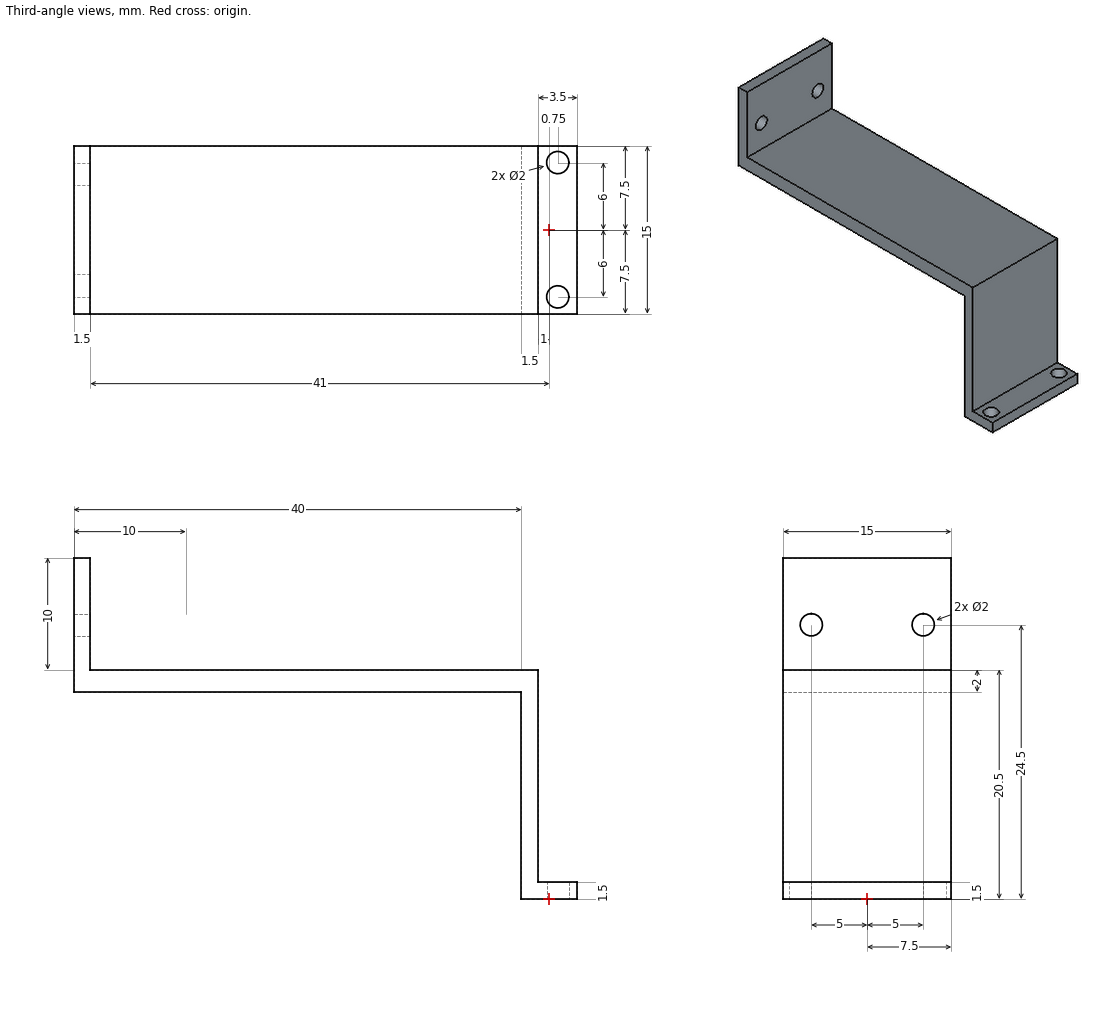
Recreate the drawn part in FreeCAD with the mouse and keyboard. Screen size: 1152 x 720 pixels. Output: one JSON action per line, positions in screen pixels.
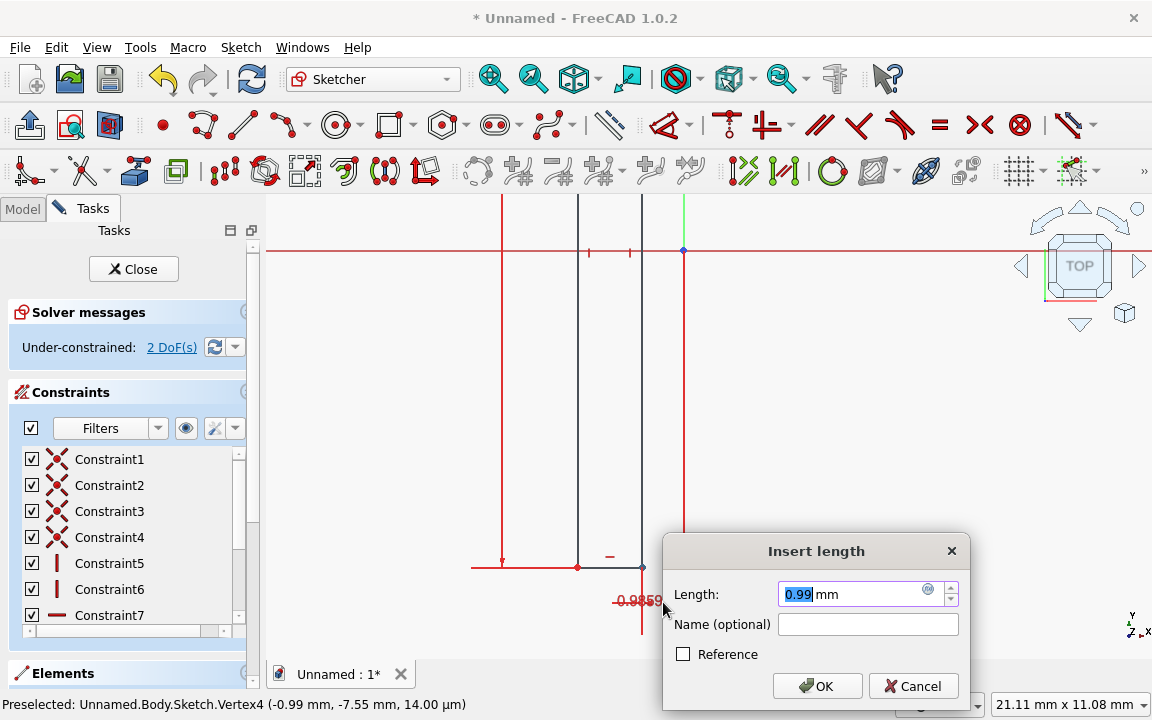
{"action": "type", "text": "1"}
{"action": "key", "text": "Return"}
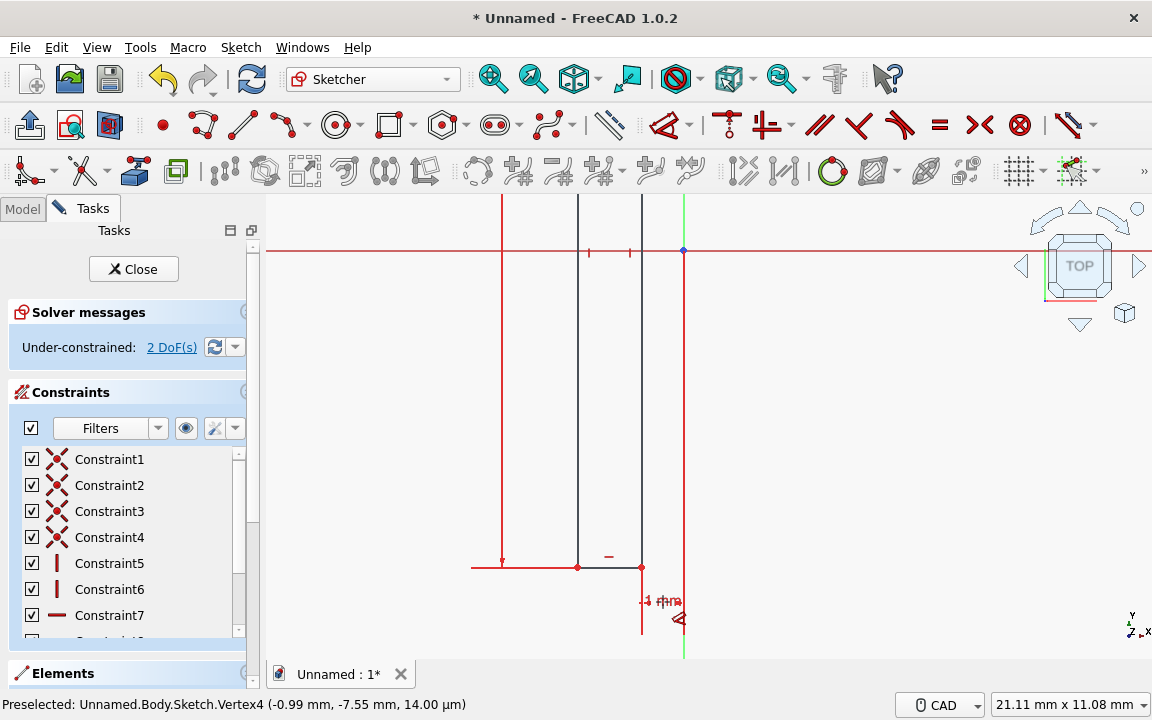
{"action": "left_click", "coordinate": [597, 568]}
{"action": "left_click", "coordinate": [588, 602]}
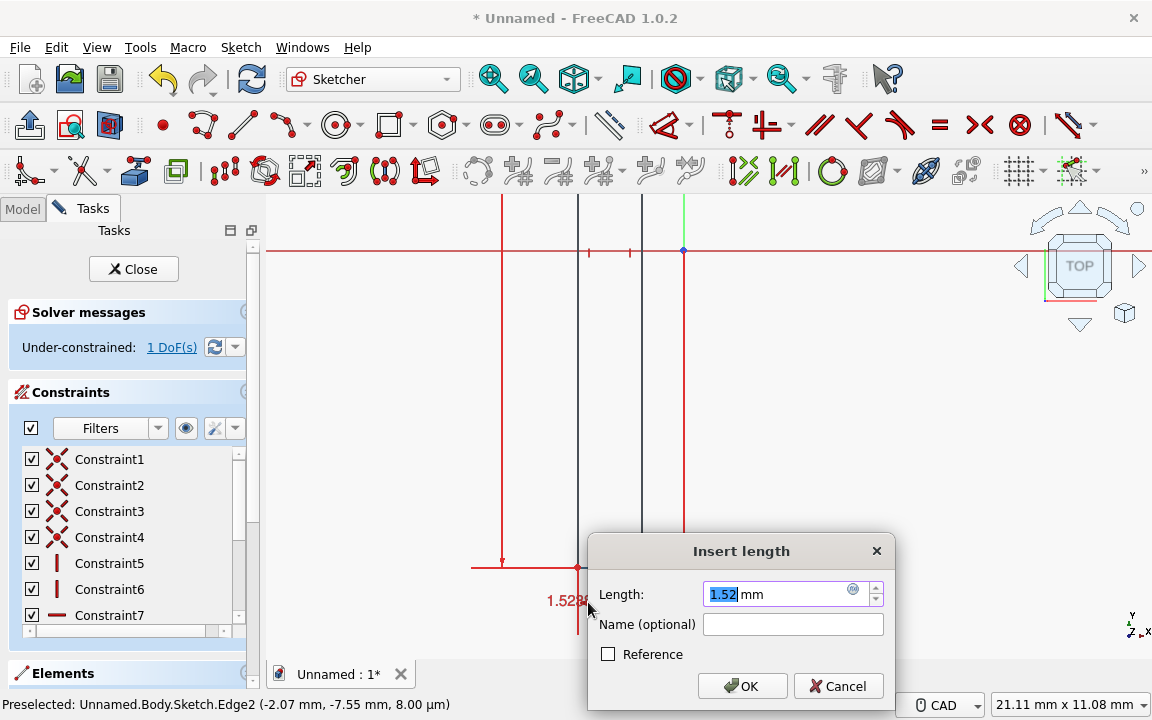
{"action": "type", "text": "1.5"}
{"action": "key", "text": "Return"}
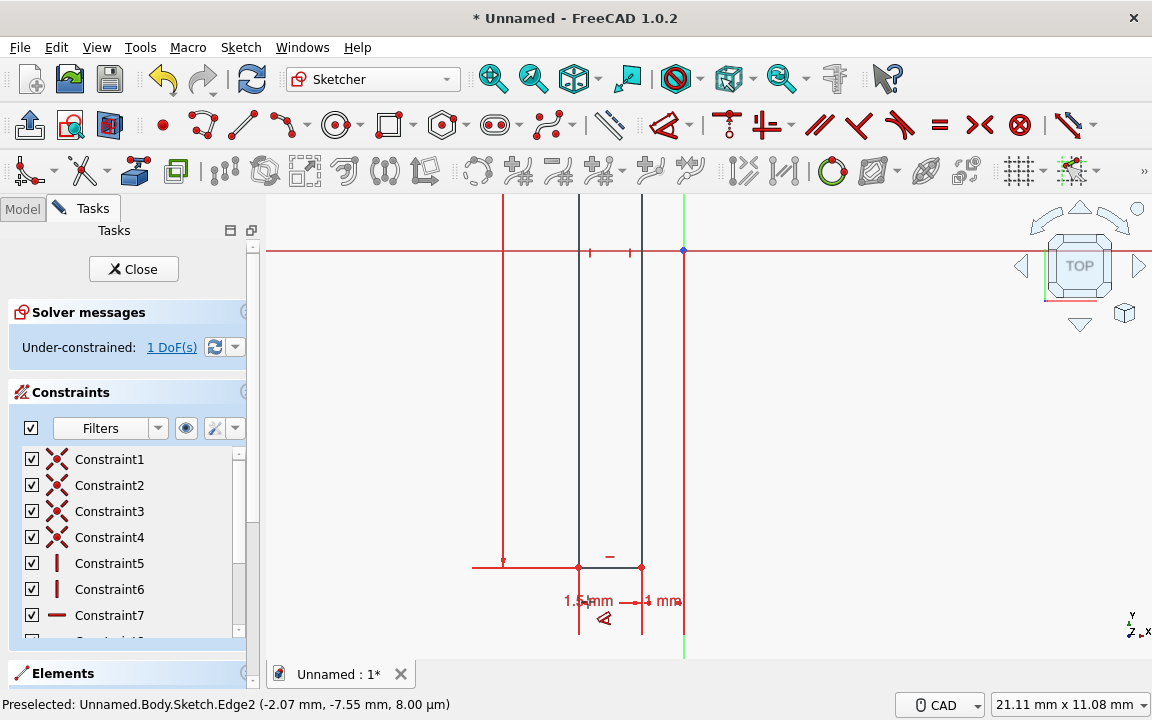
{"action": "scroll", "coordinate": [648, 570], "scroll_direction": "down", "scroll_amount": 4}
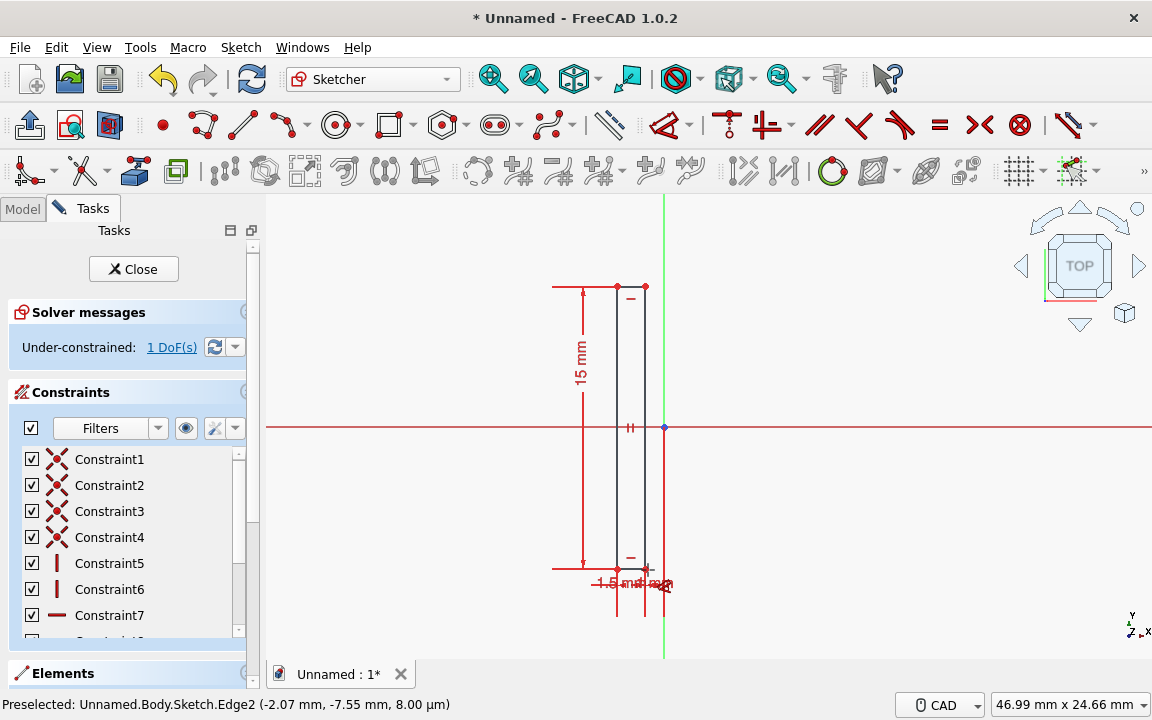
{"action": "left_click", "coordinate": [617, 287]}
{"action": "left_click", "coordinate": [698, 357]}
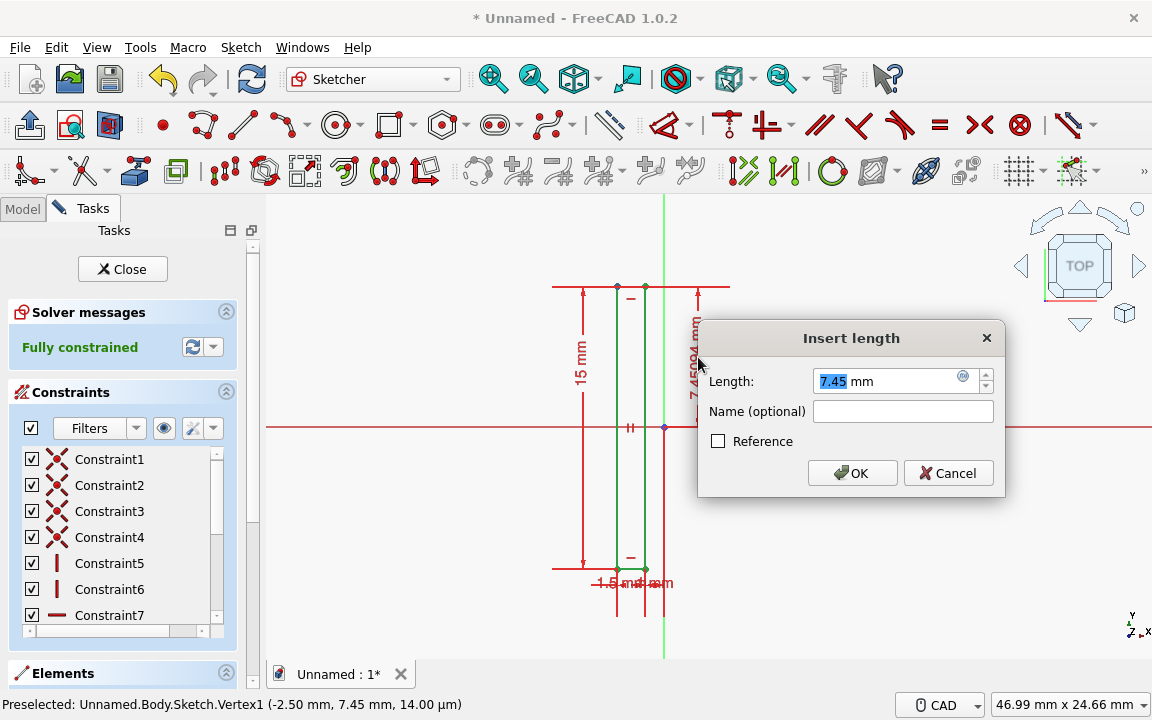
{"action": "type", "text": "7.5"}
{"action": "key", "text": "Return"}
{"action": "key", "text": "Escape"}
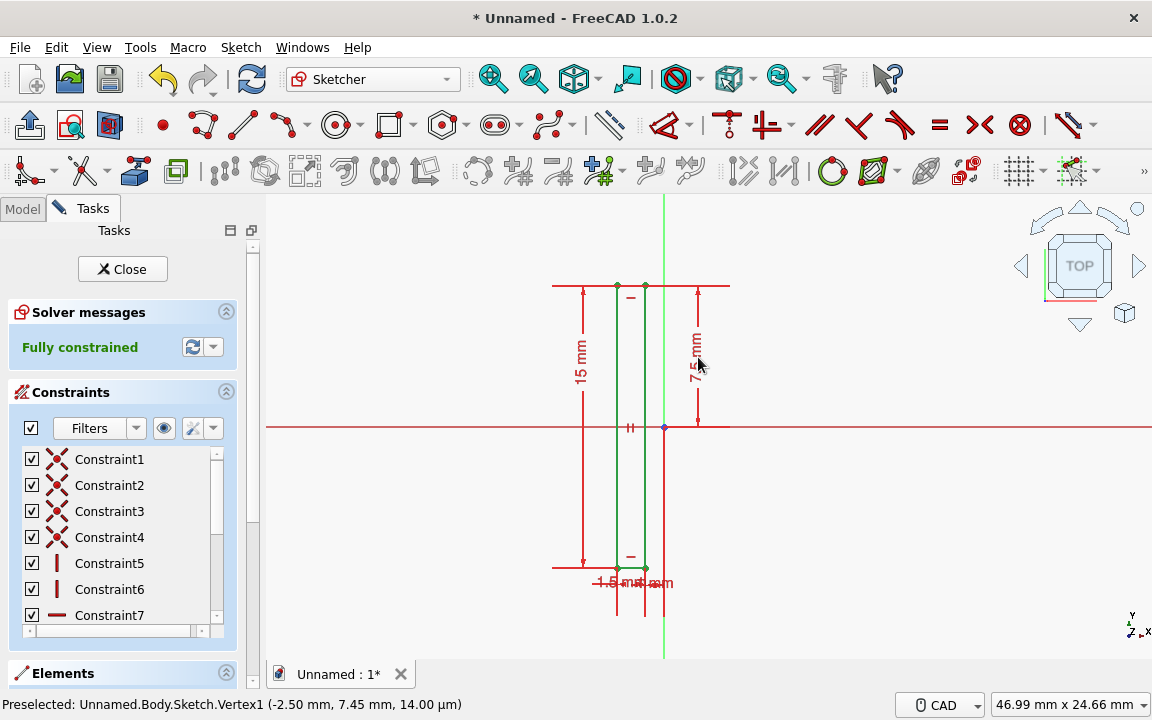
{"action": "left_click", "coordinate": [123, 269]}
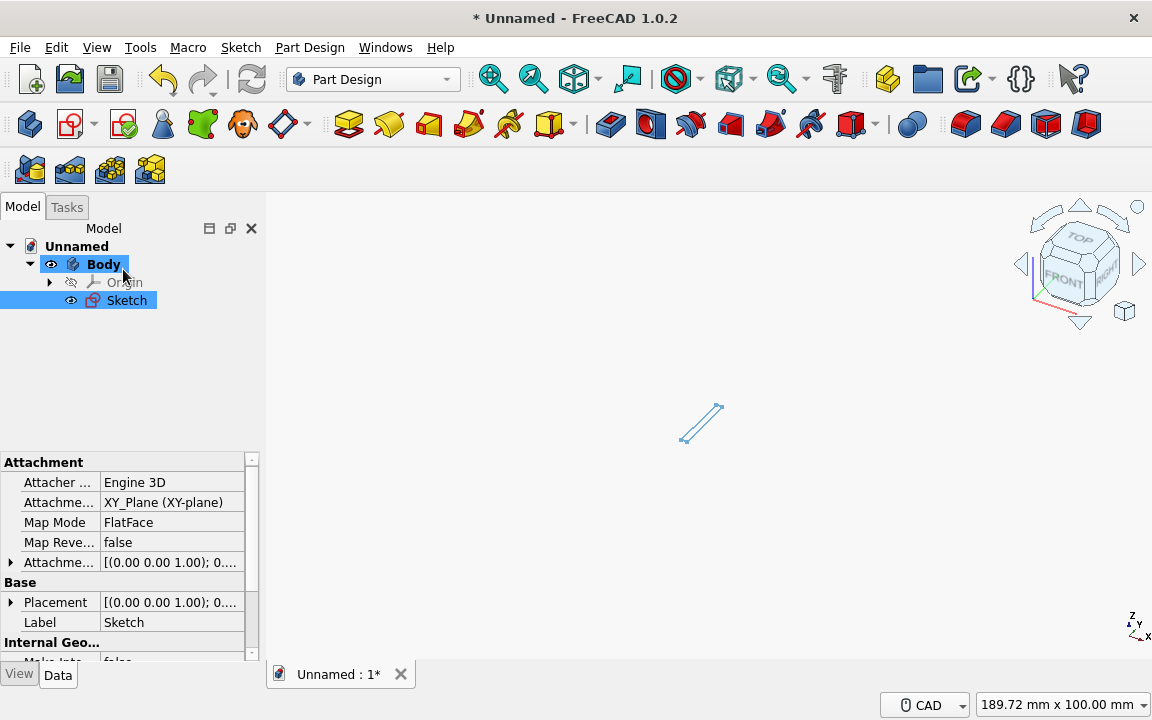
{"action": "left_click", "coordinate": [350, 124]}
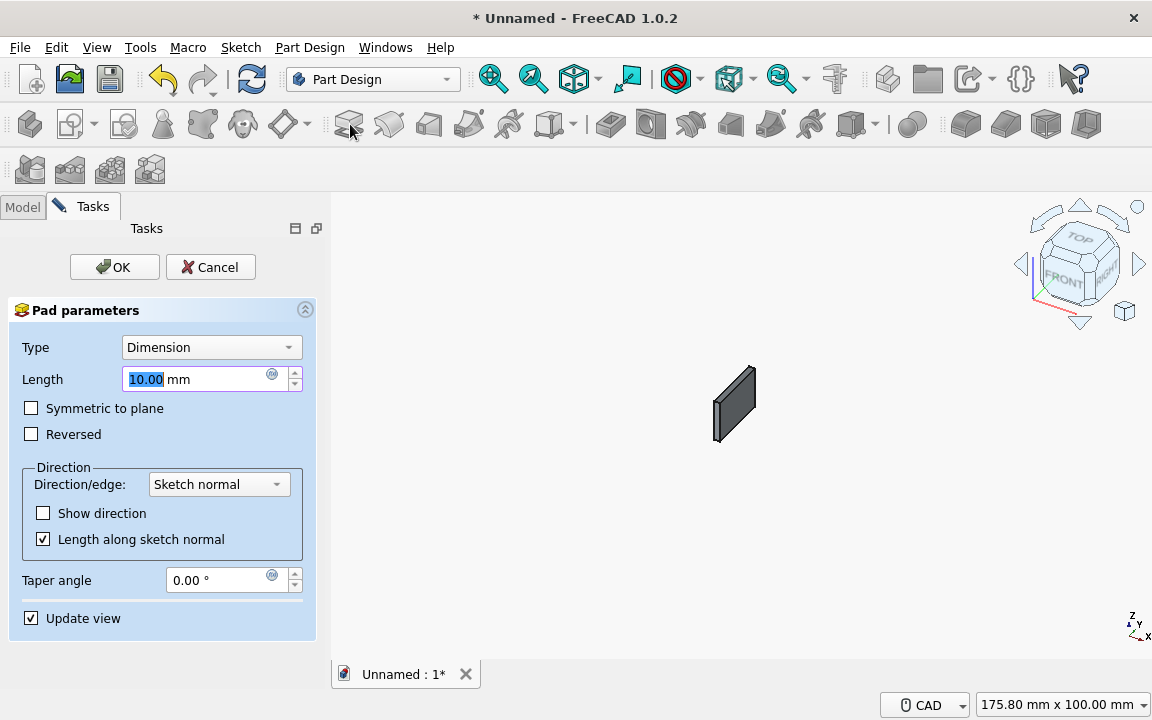
{"action": "type", "text": "20.5"}
{"action": "key", "text": "Tab"}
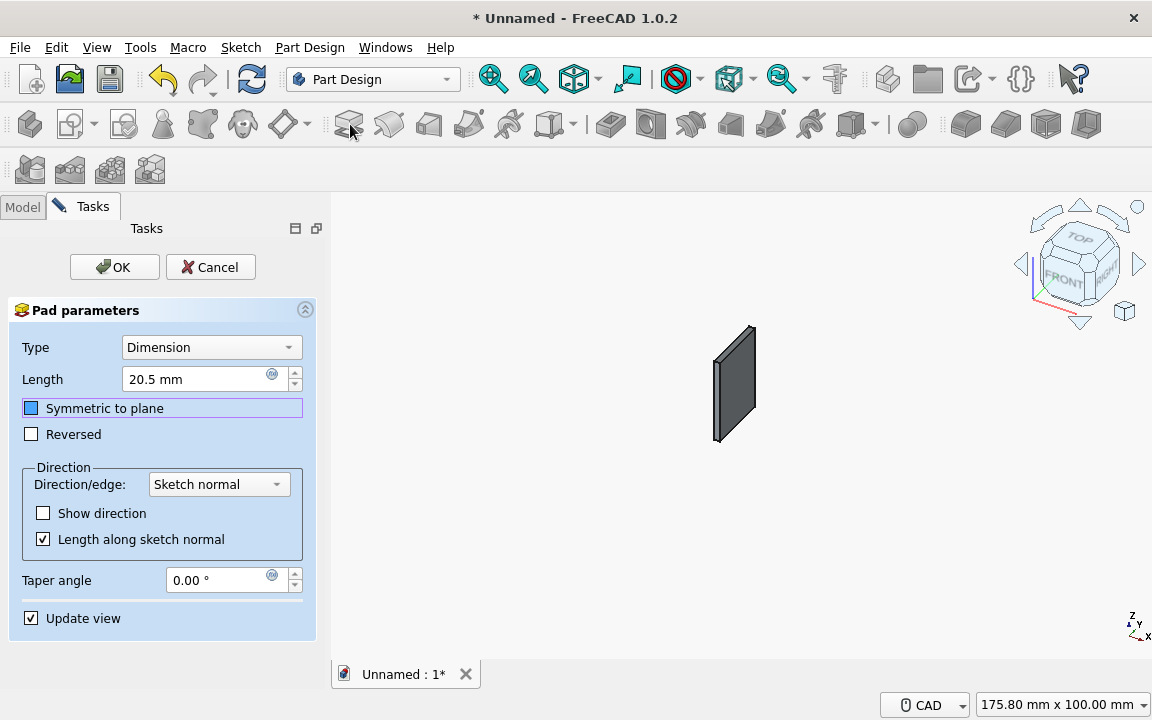
{"action": "left_click", "coordinate": [115, 267]}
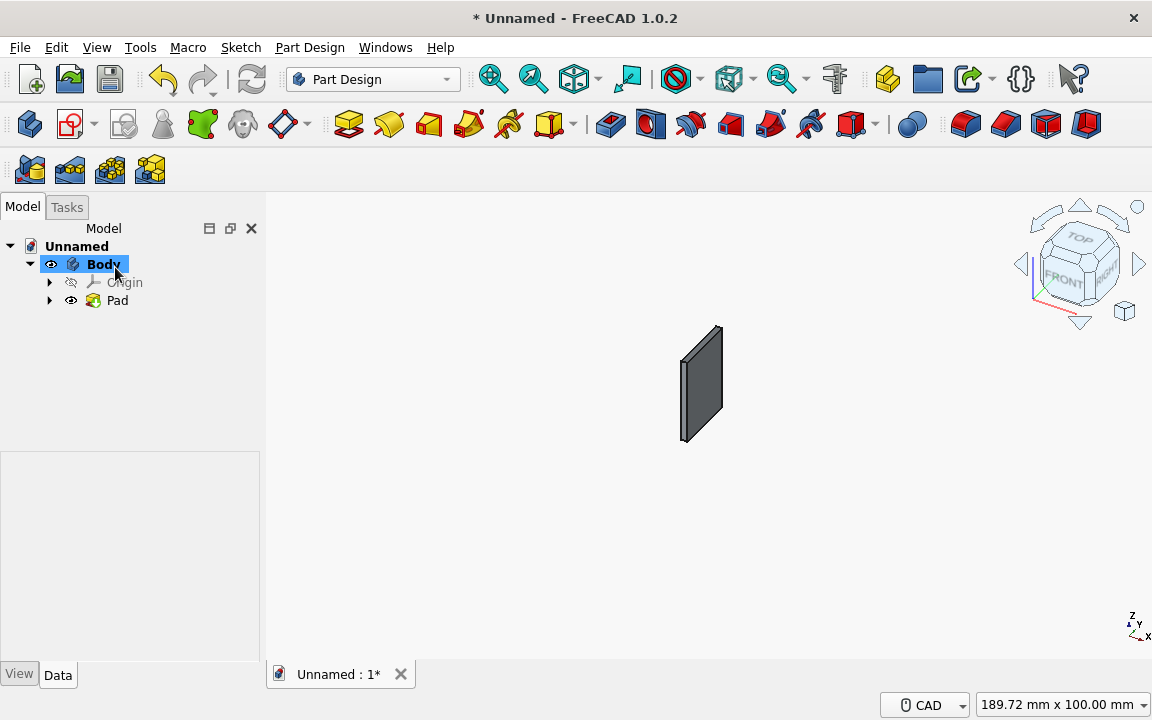
{"action": "key", "text": "v f"}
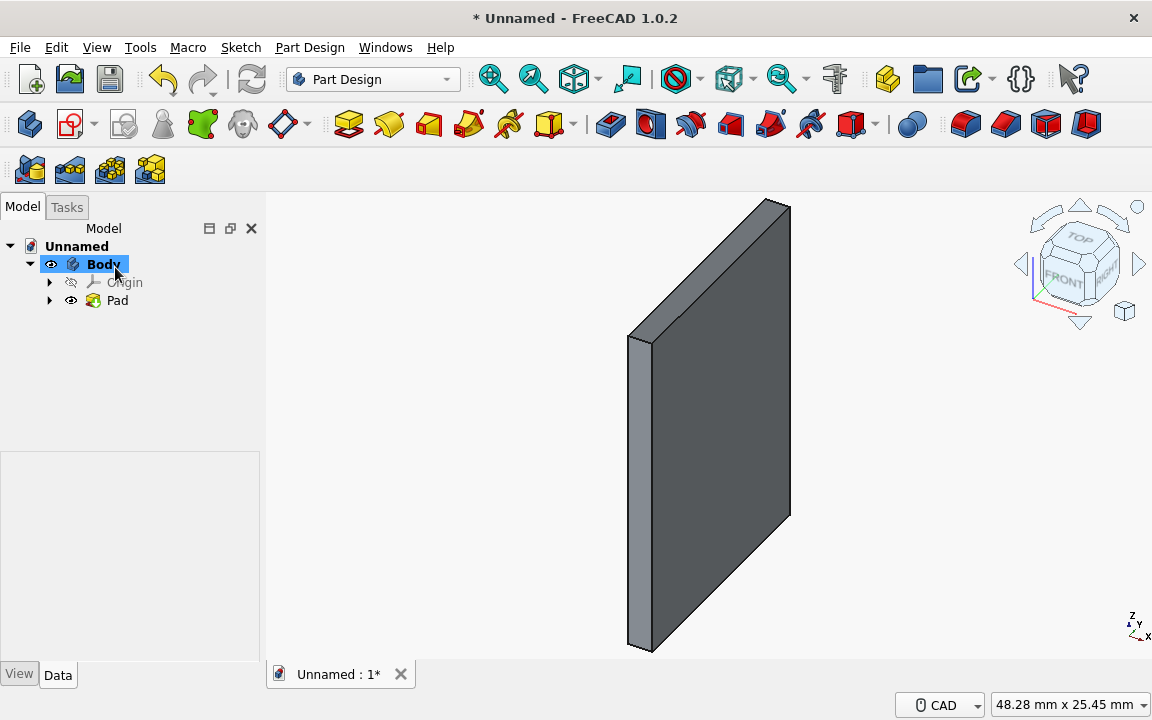
{"action": "key", "text": "5"}